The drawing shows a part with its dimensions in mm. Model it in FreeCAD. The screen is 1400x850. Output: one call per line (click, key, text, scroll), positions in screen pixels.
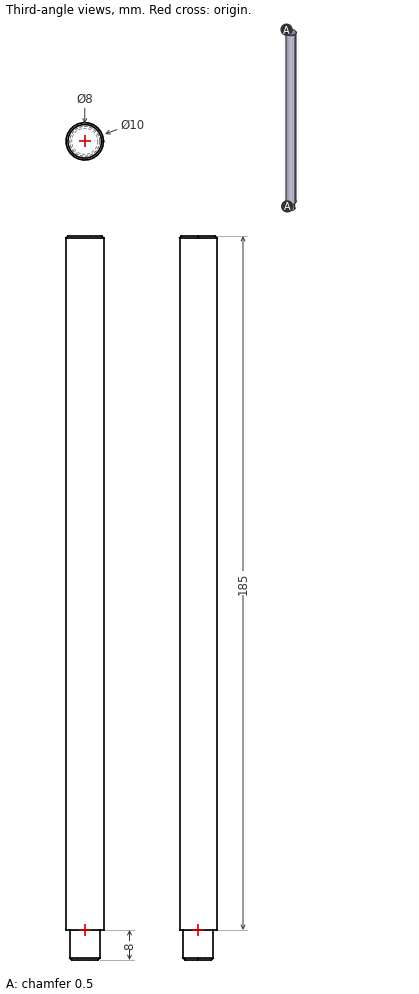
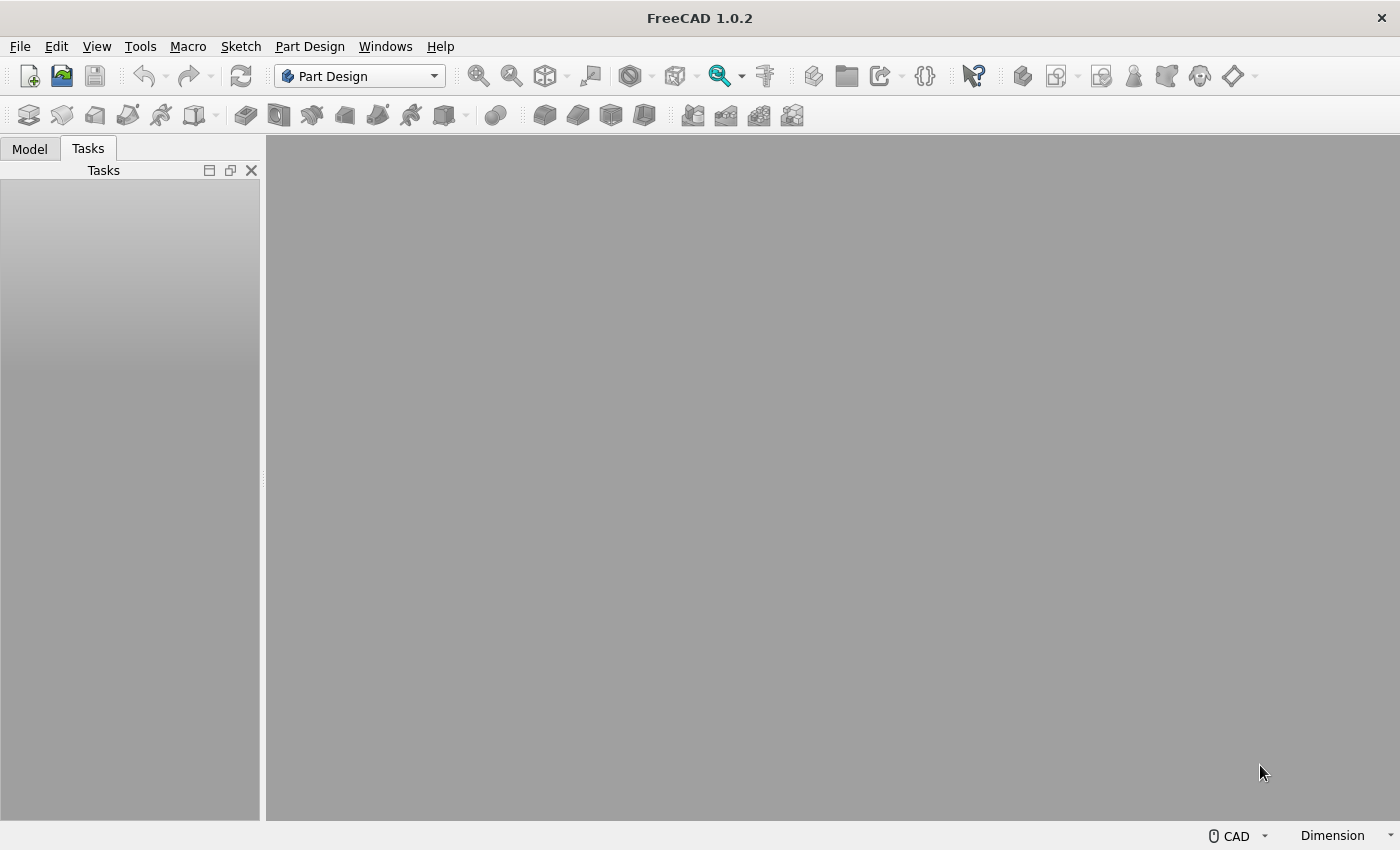
key(ctrl+n)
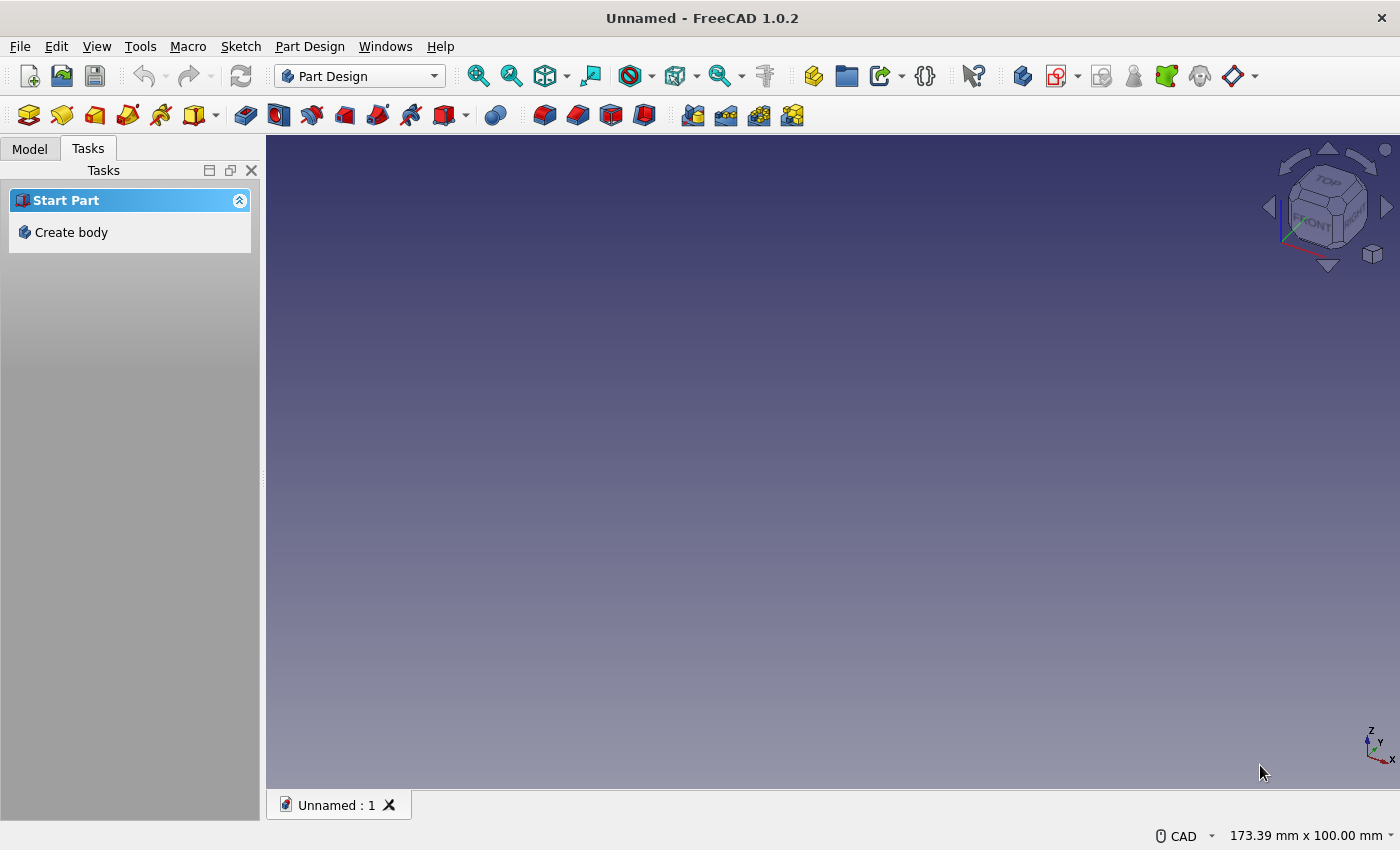
click(1056, 76)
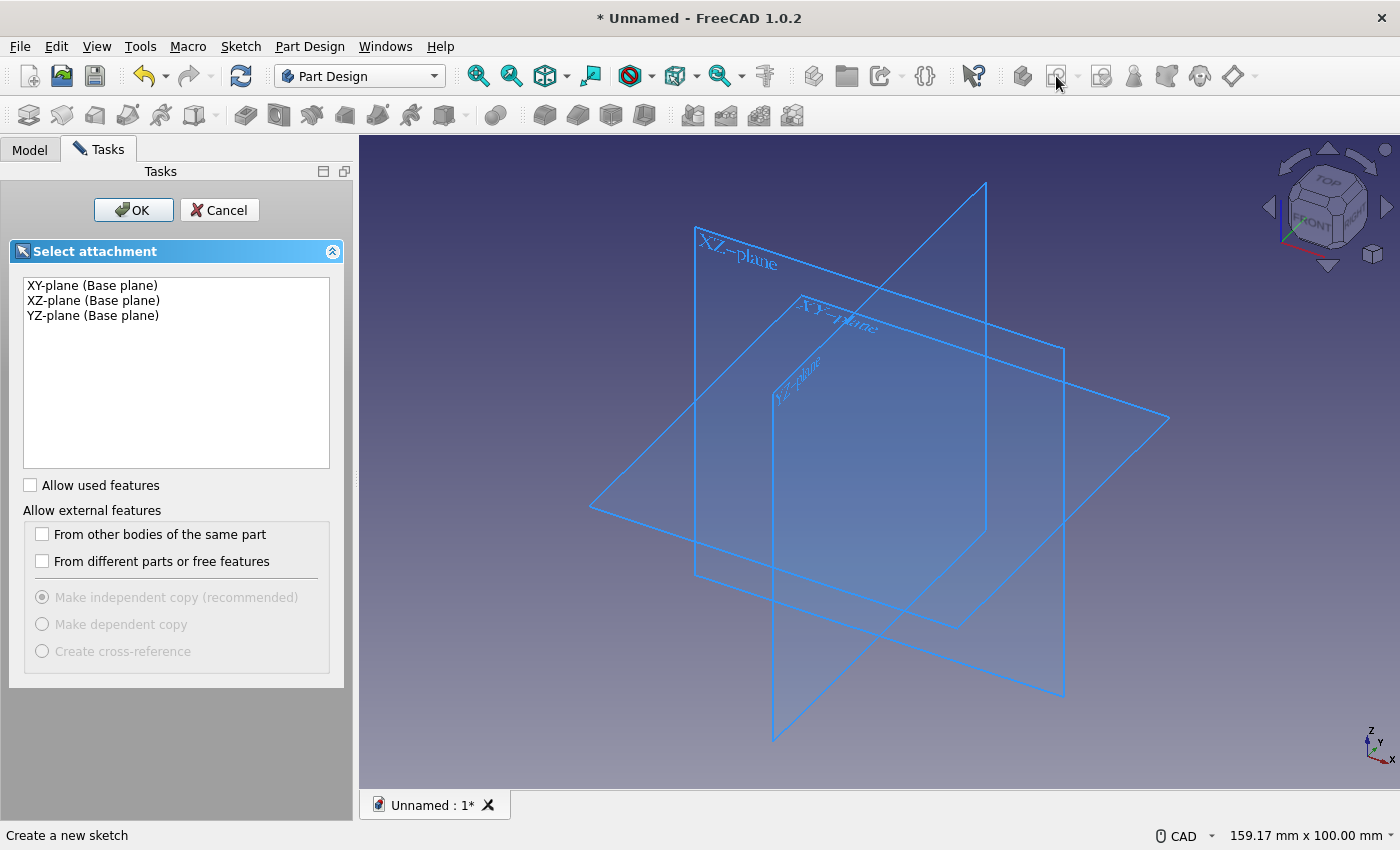
click(84, 286)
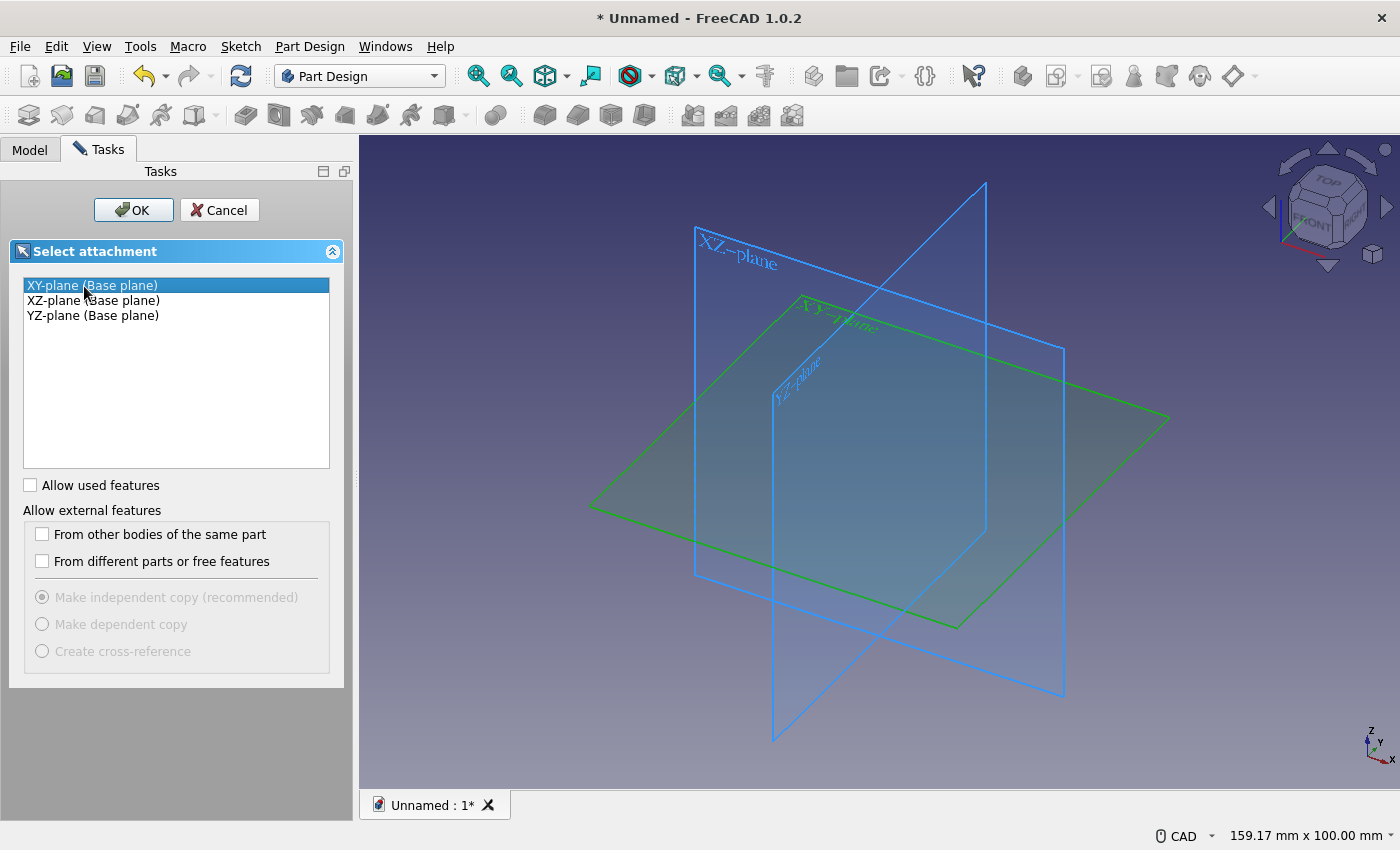
click(134, 210)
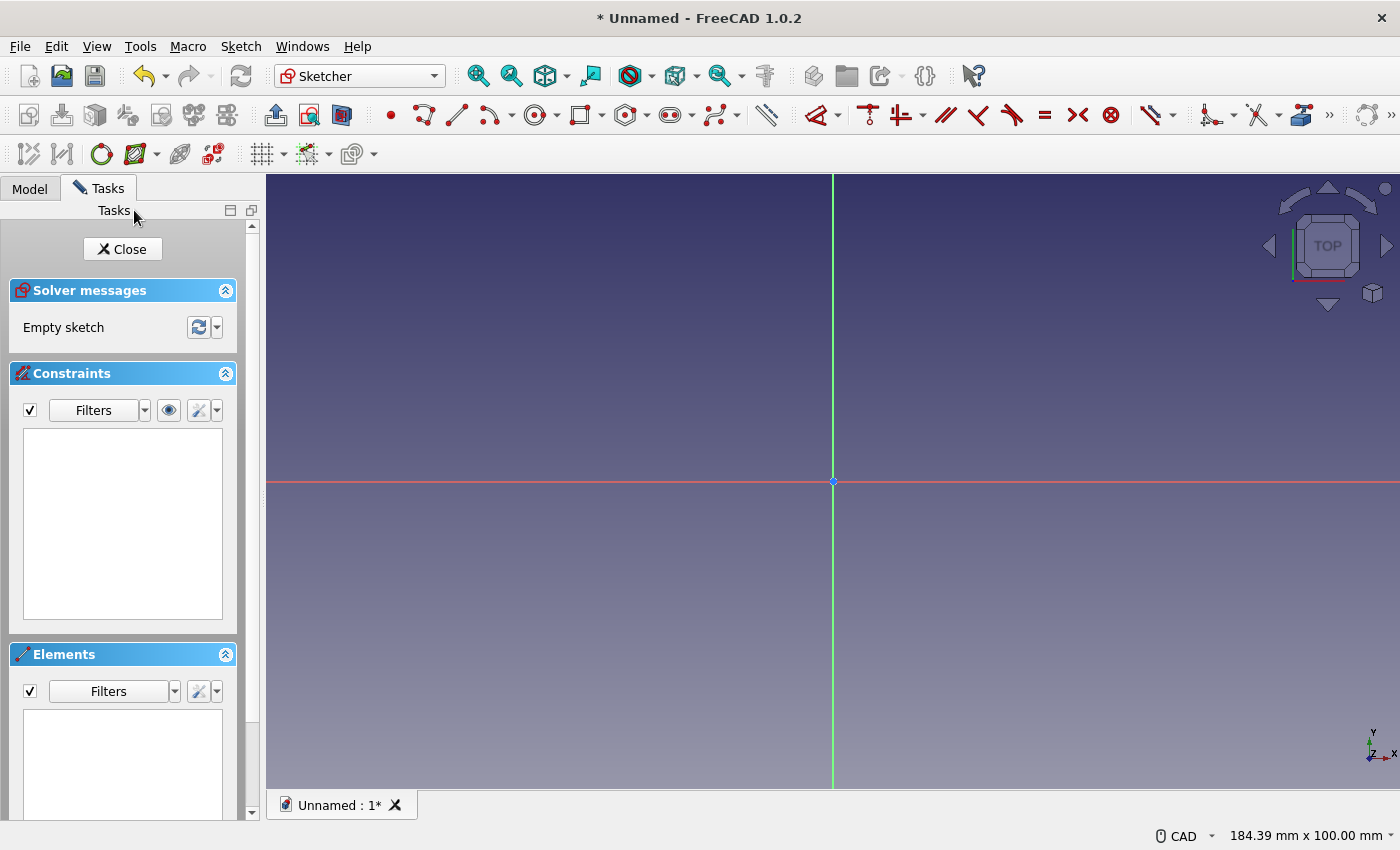
scroll(847, 482, up, 9)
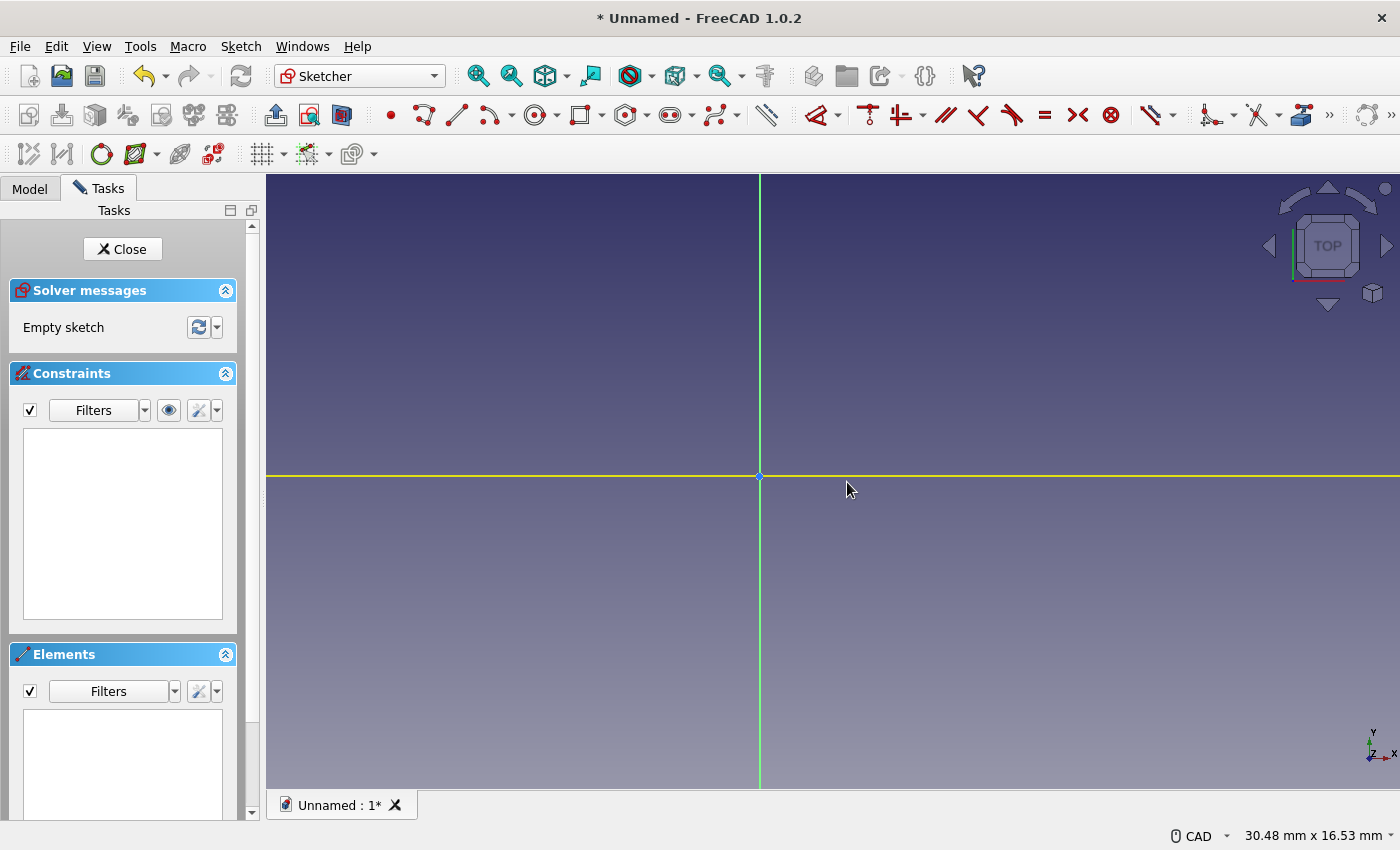
click(534, 116)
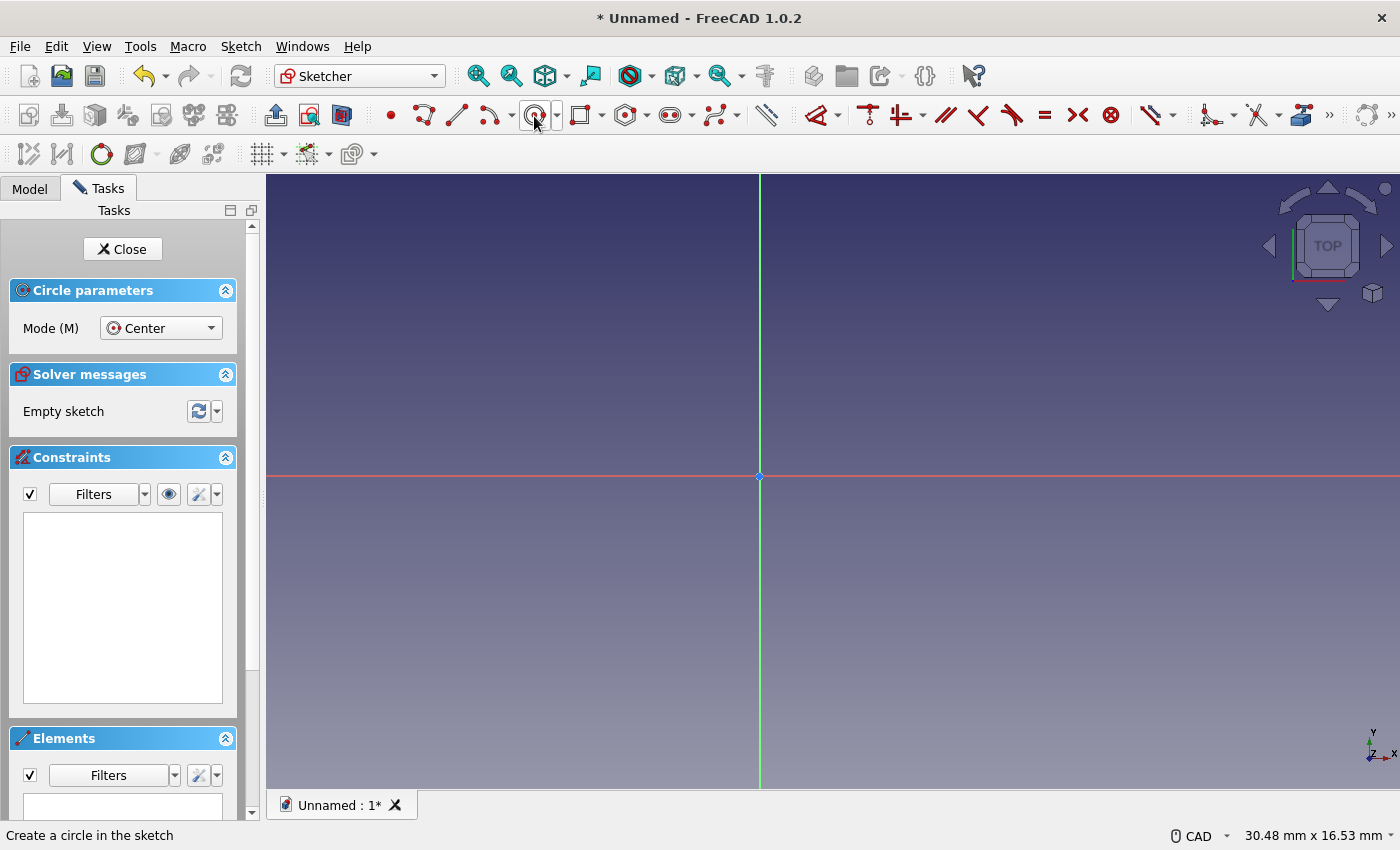
click(760, 476)
click(891, 345)
key(Escape)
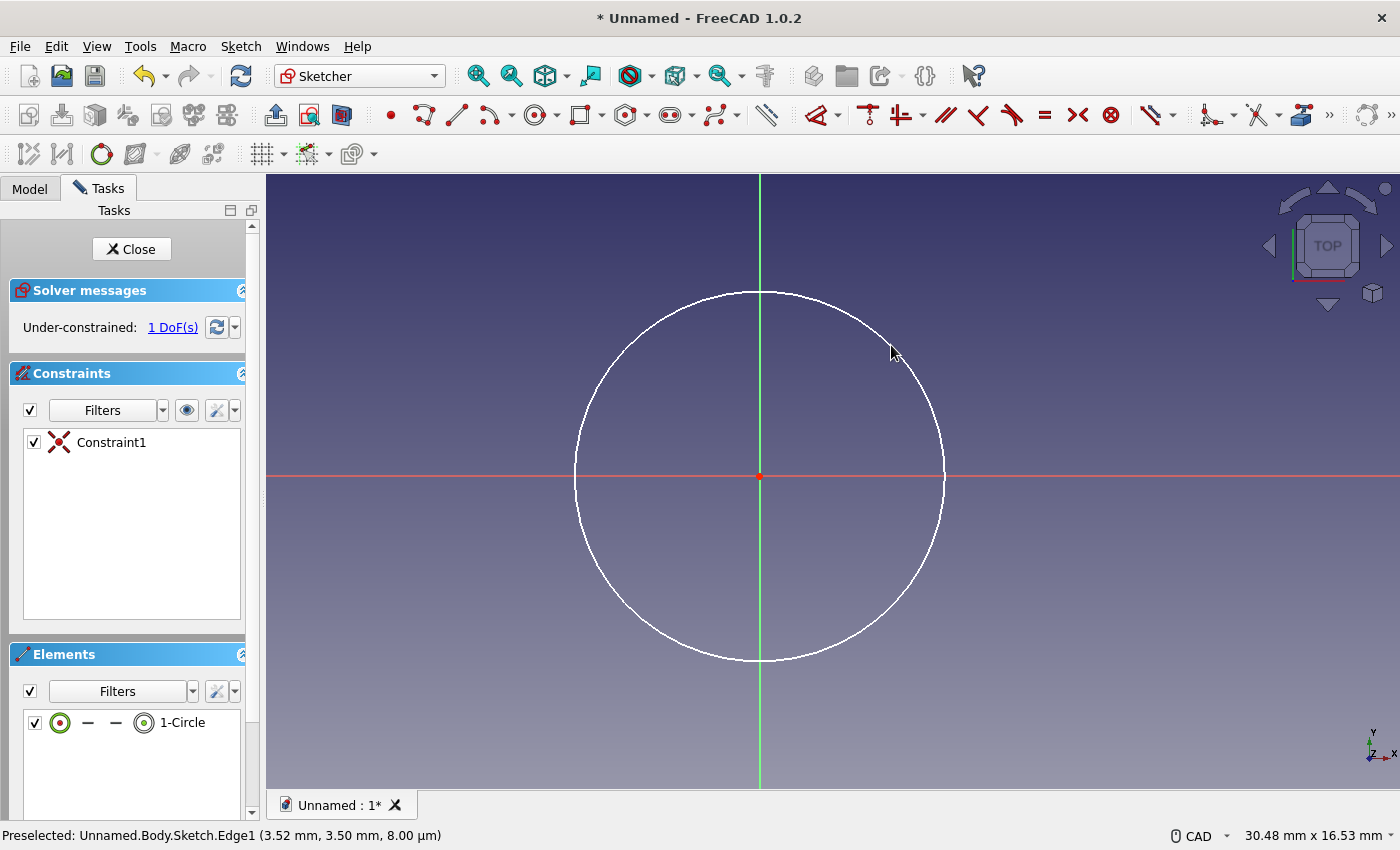
click(890, 345)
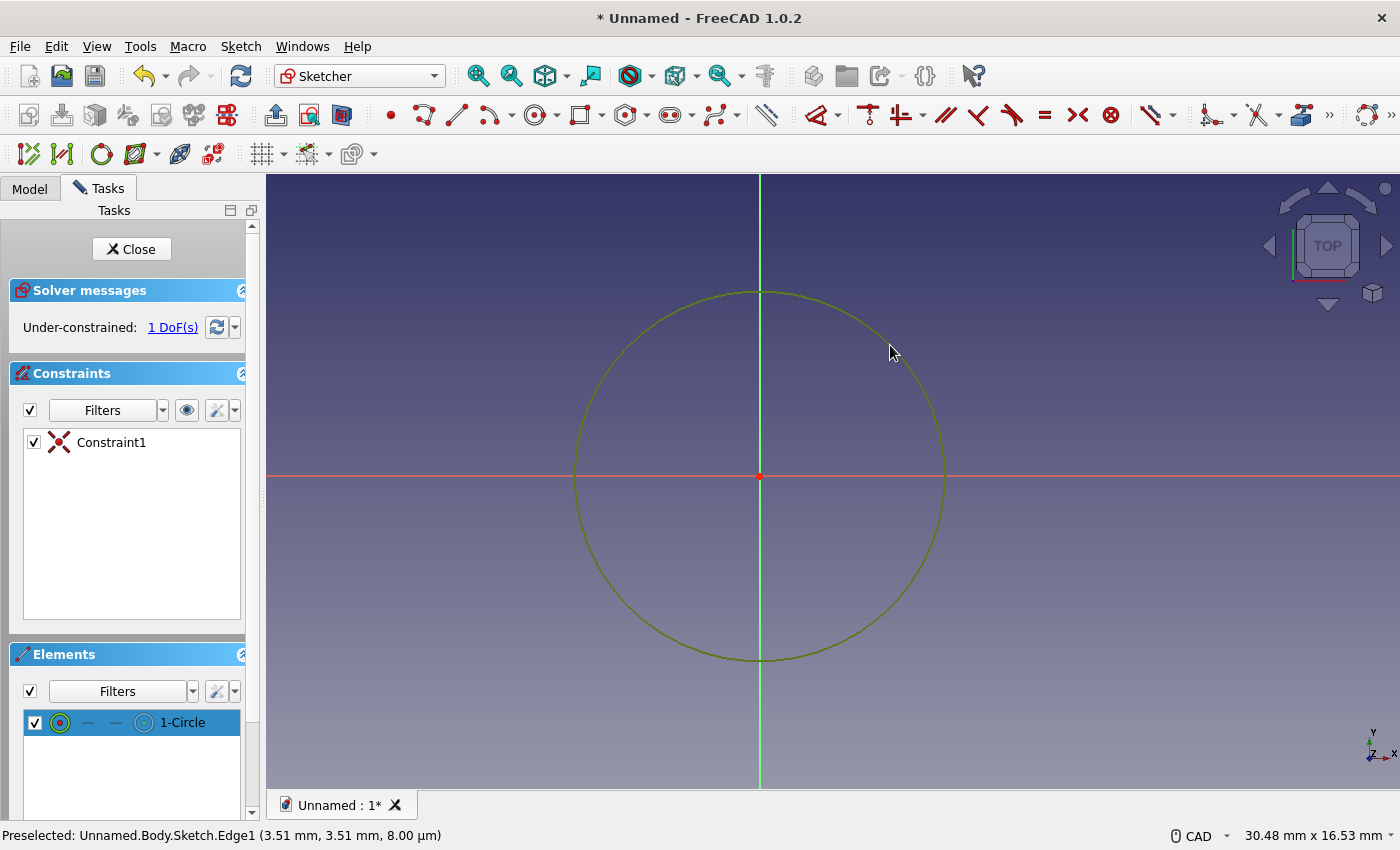
key(k)
key(o)